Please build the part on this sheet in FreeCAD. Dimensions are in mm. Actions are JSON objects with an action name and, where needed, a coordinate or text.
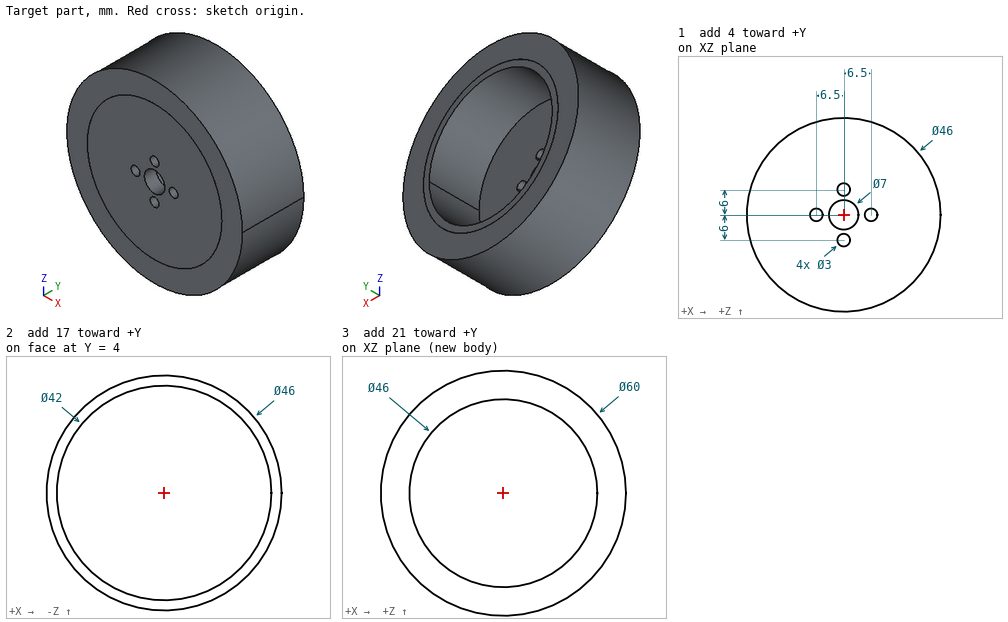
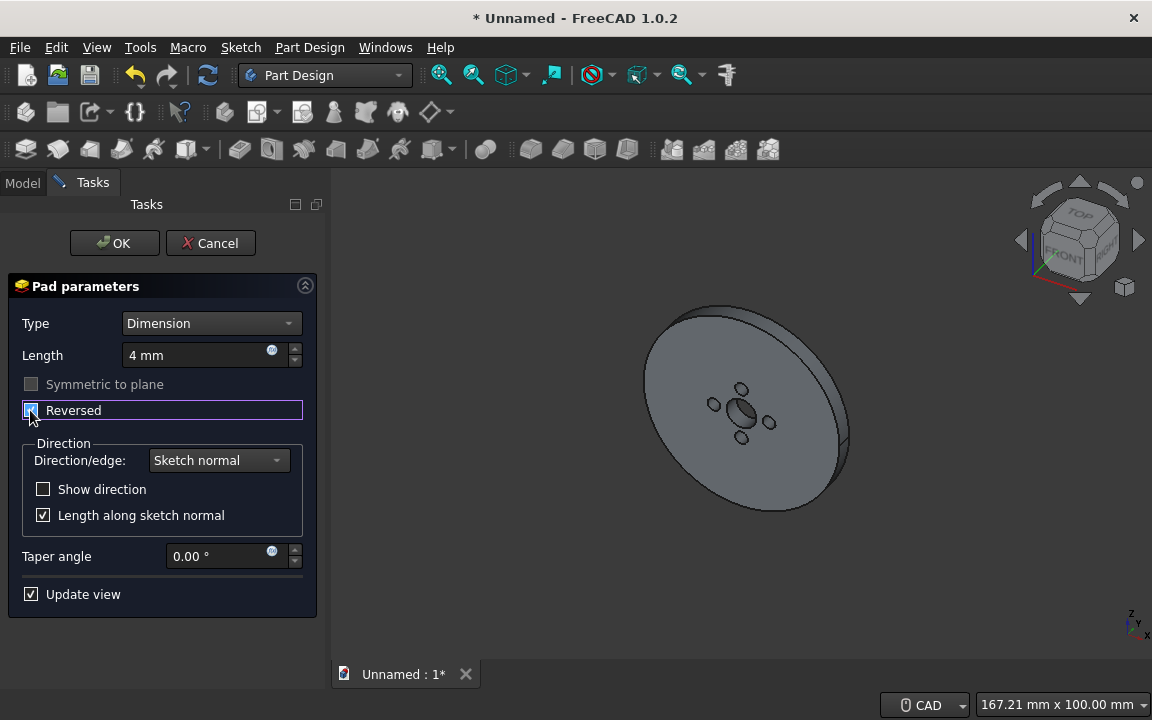
{"action": "left_click", "coordinate": [115, 243]}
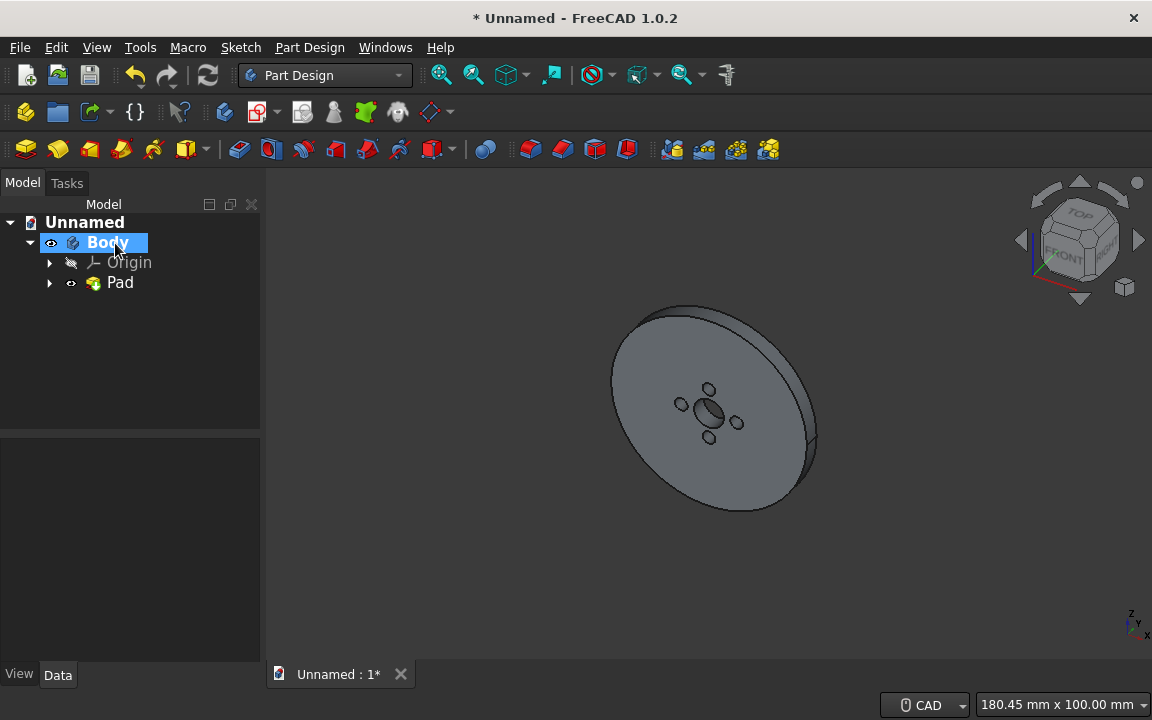
{"action": "key", "text": "4"}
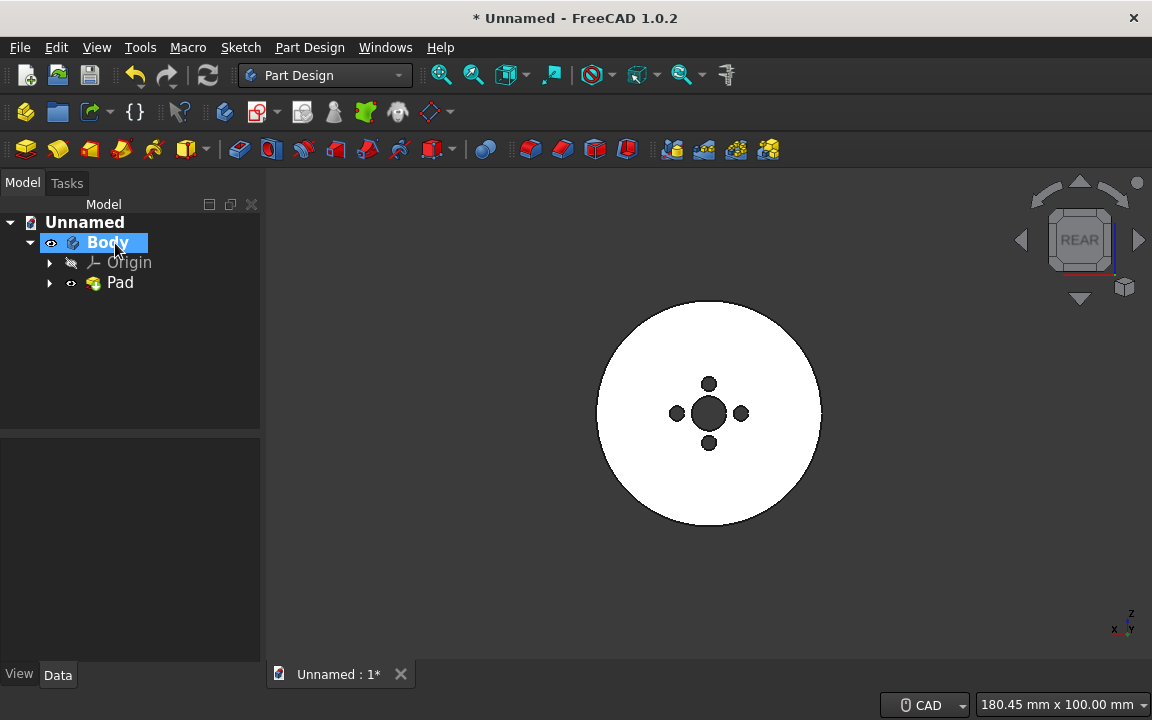
{"action": "left_click", "coordinate": [741, 348]}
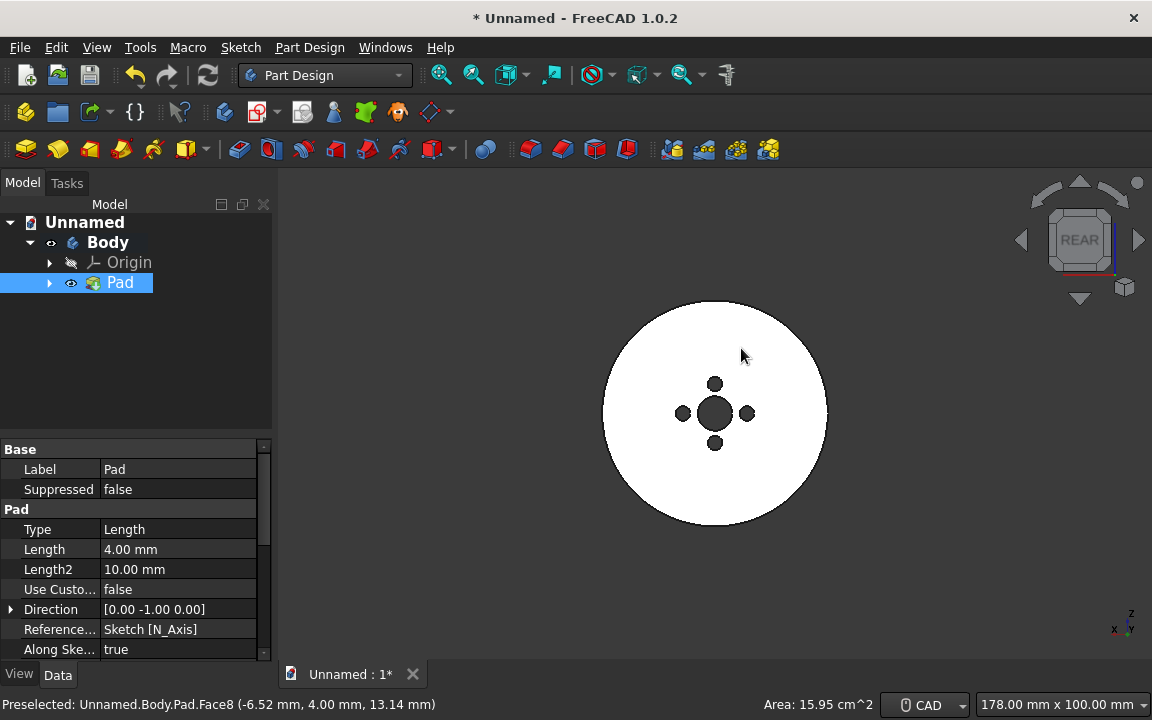
{"action": "left_click", "coordinate": [258, 112]}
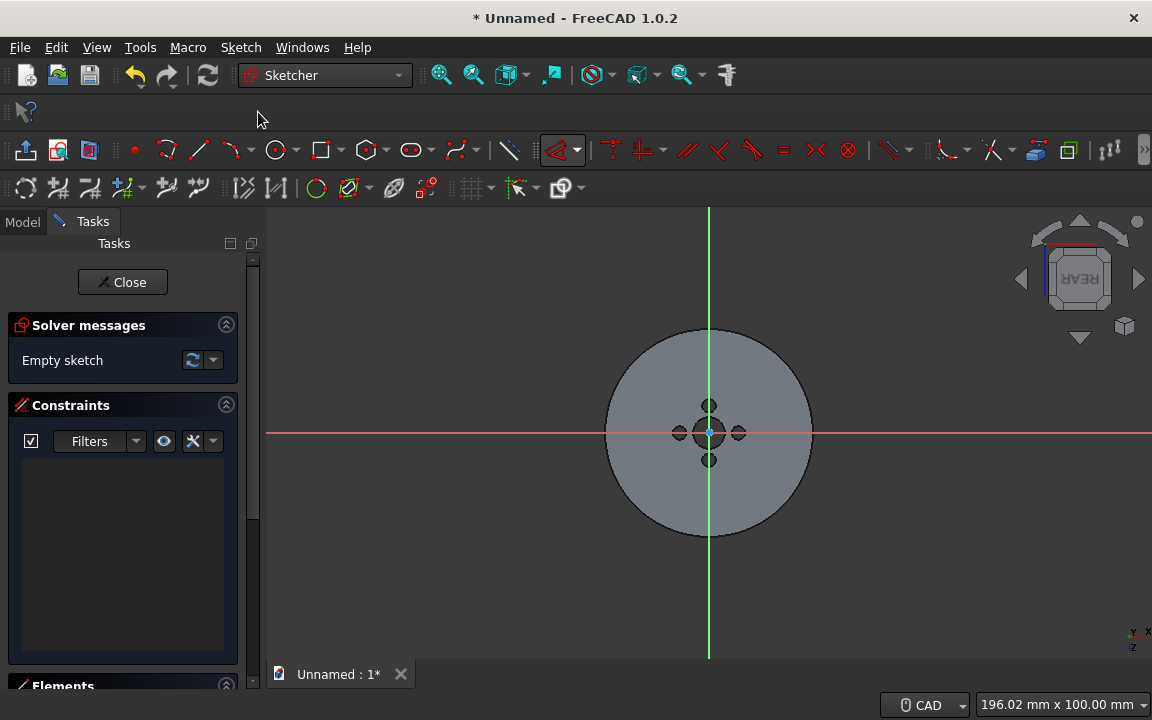
{"action": "left_click", "coordinate": [276, 150]}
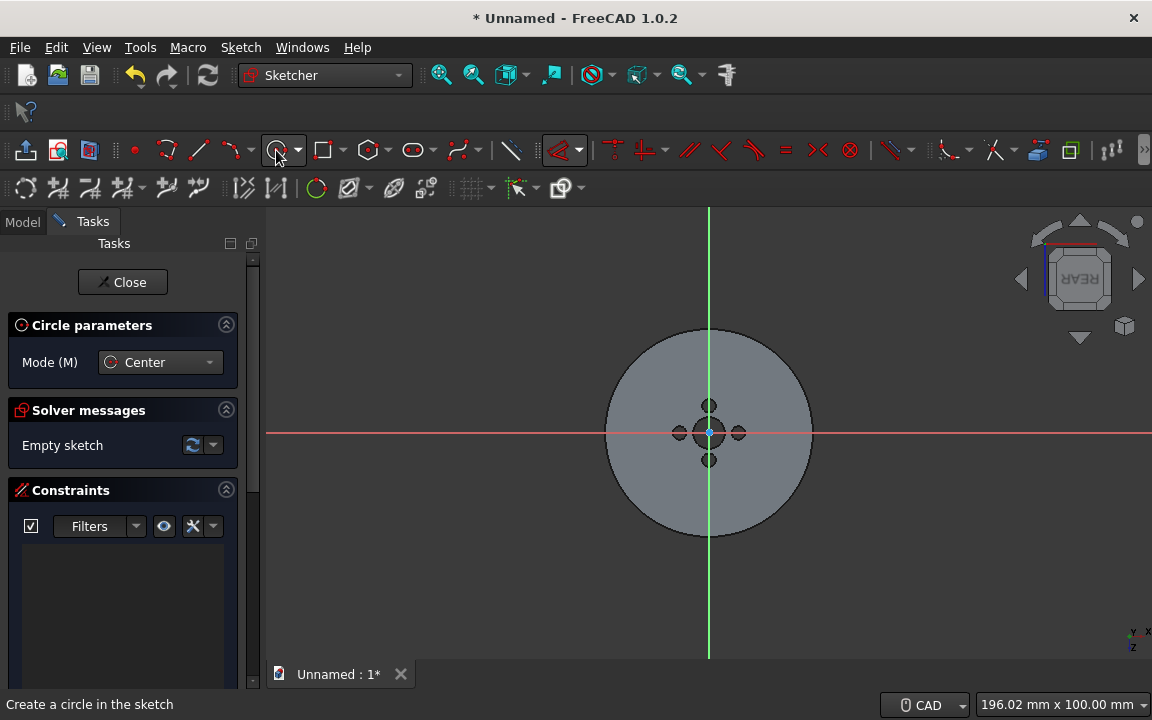
{"action": "left_click", "coordinate": [709, 433]}
{"action": "left_click", "coordinate": [783, 359]}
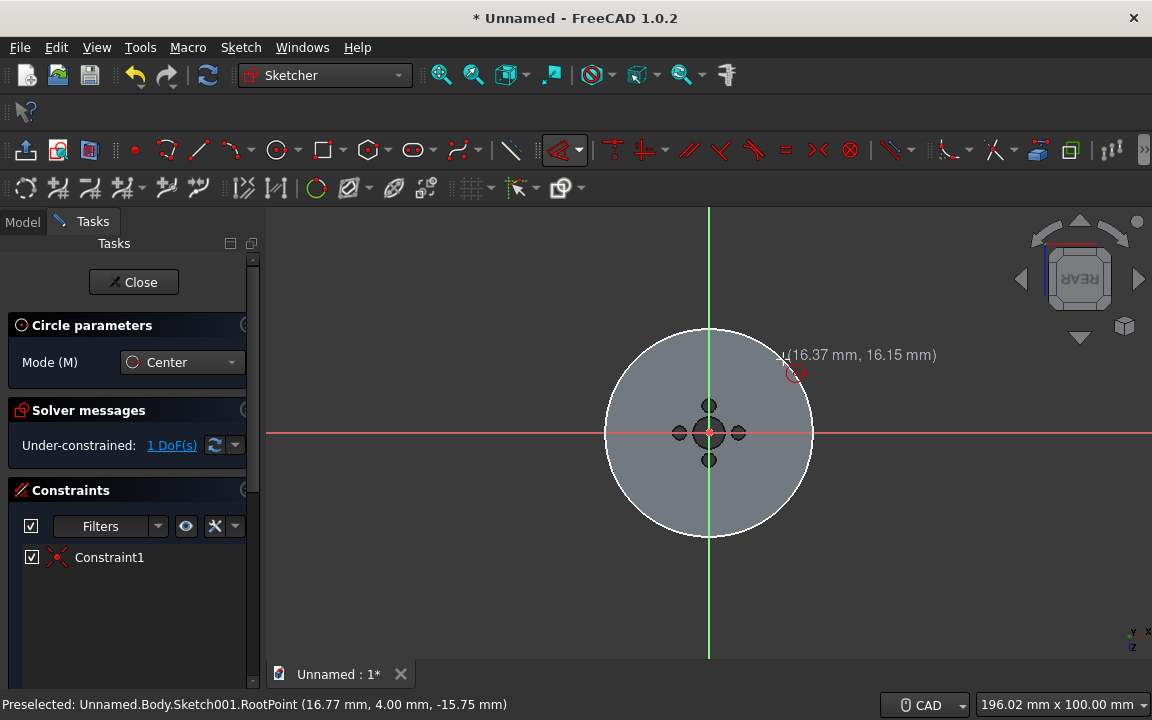
{"action": "left_click", "coordinate": [709, 433]}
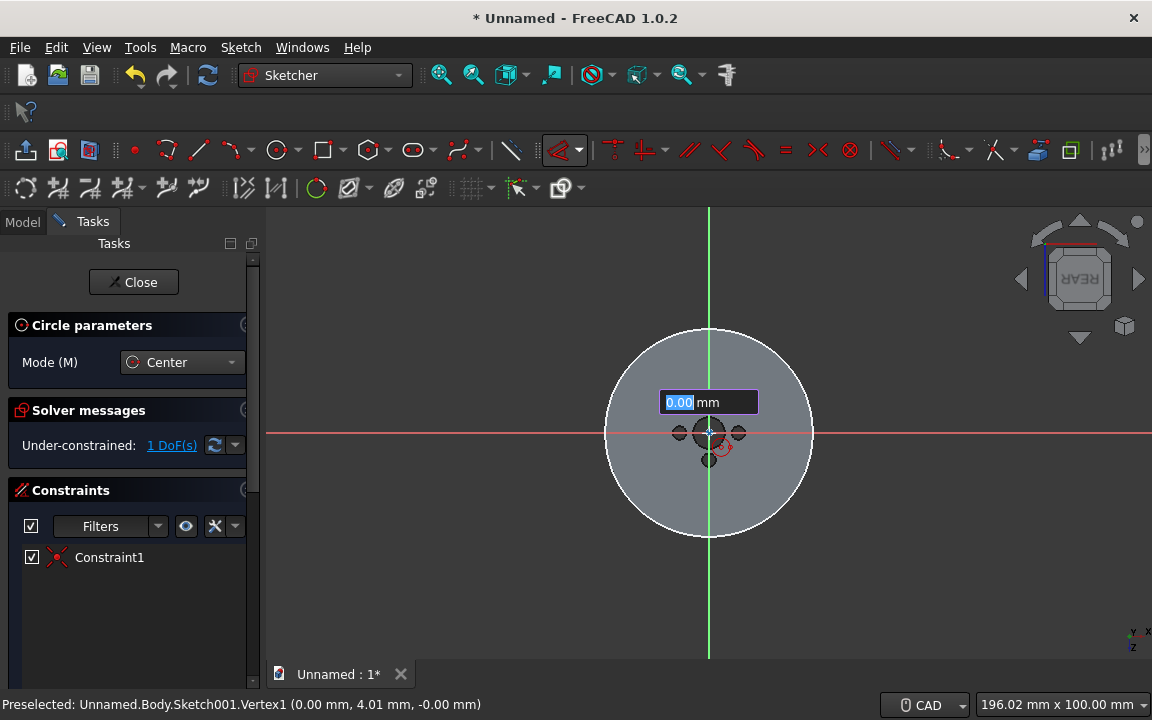
{"action": "scroll", "coordinate": [776, 366], "scroll_direction": "up", "scroll_amount": 3}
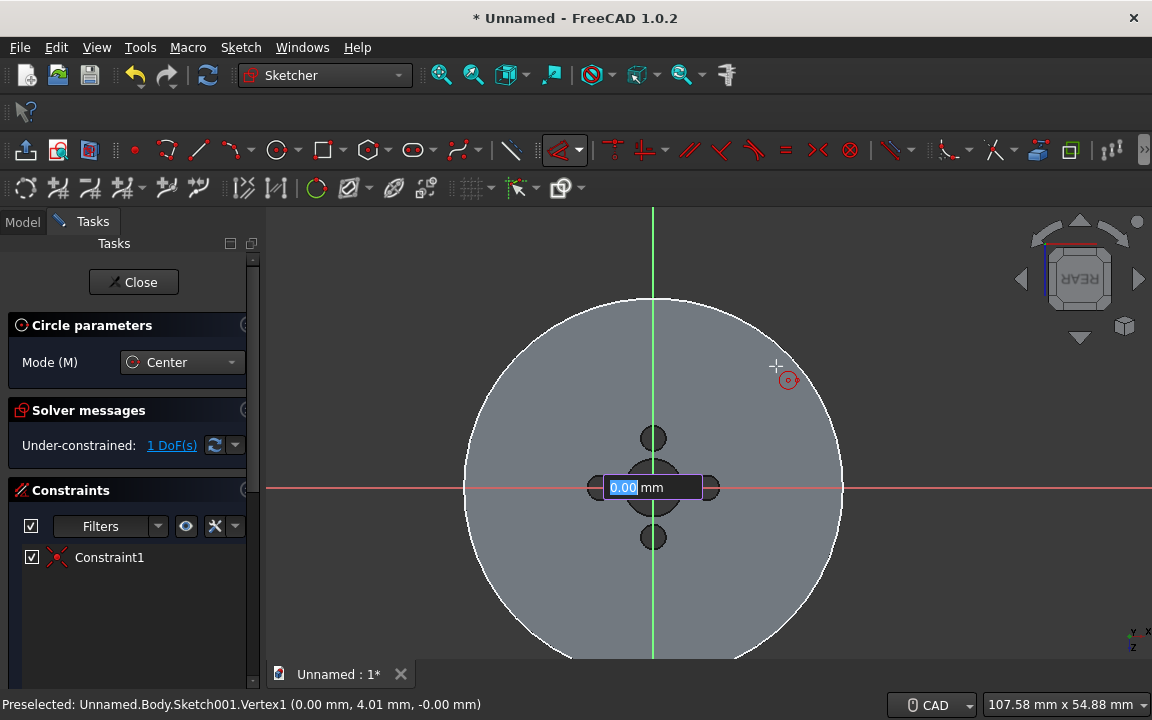
{"action": "left_click", "coordinate": [776, 365]}
{"action": "key", "text": "Escape"}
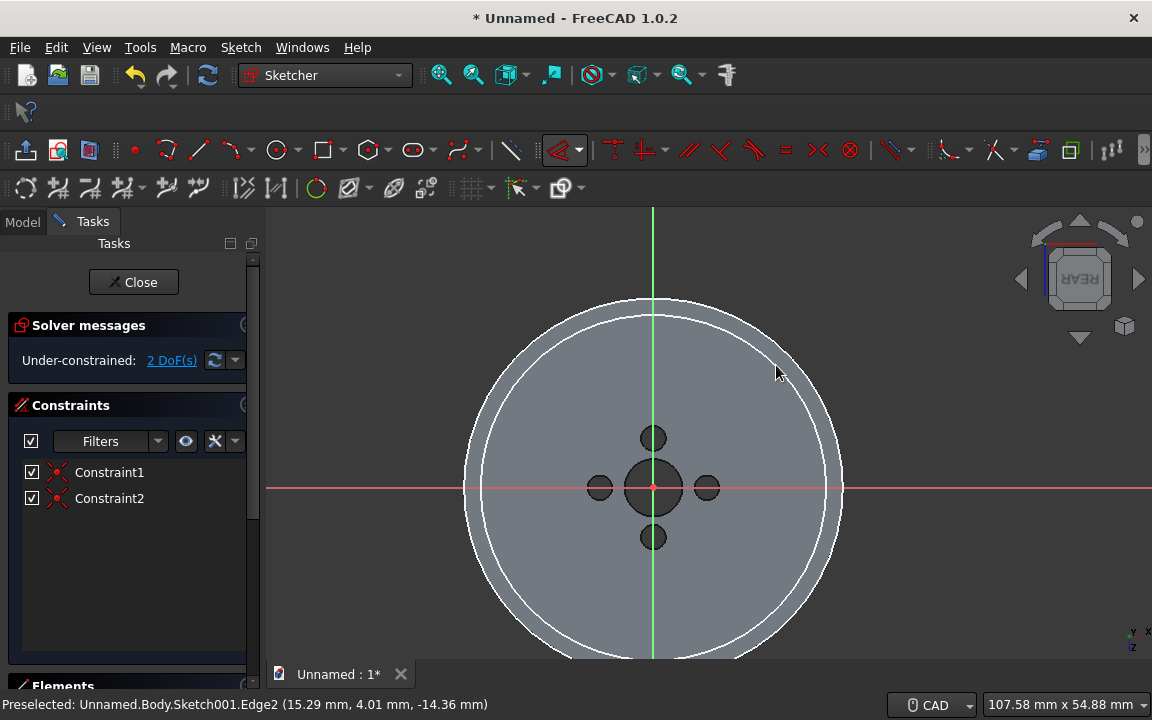
{"action": "left_click", "coordinate": [787, 353]}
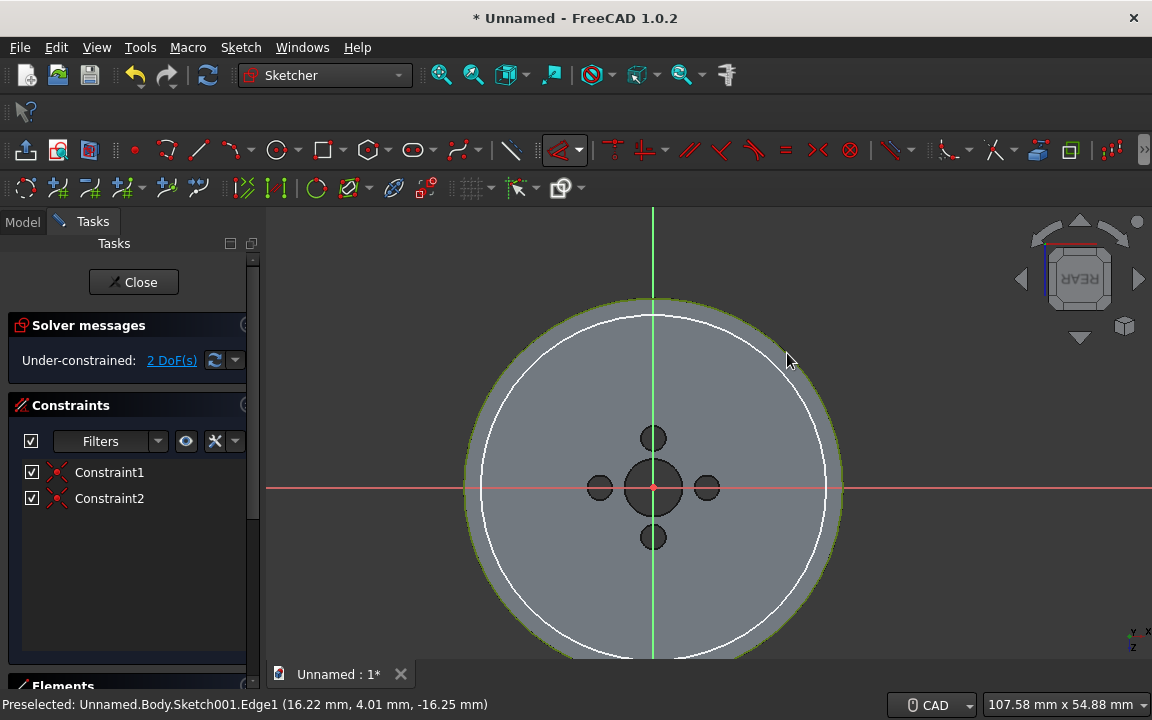
{"action": "key", "text": "k o"}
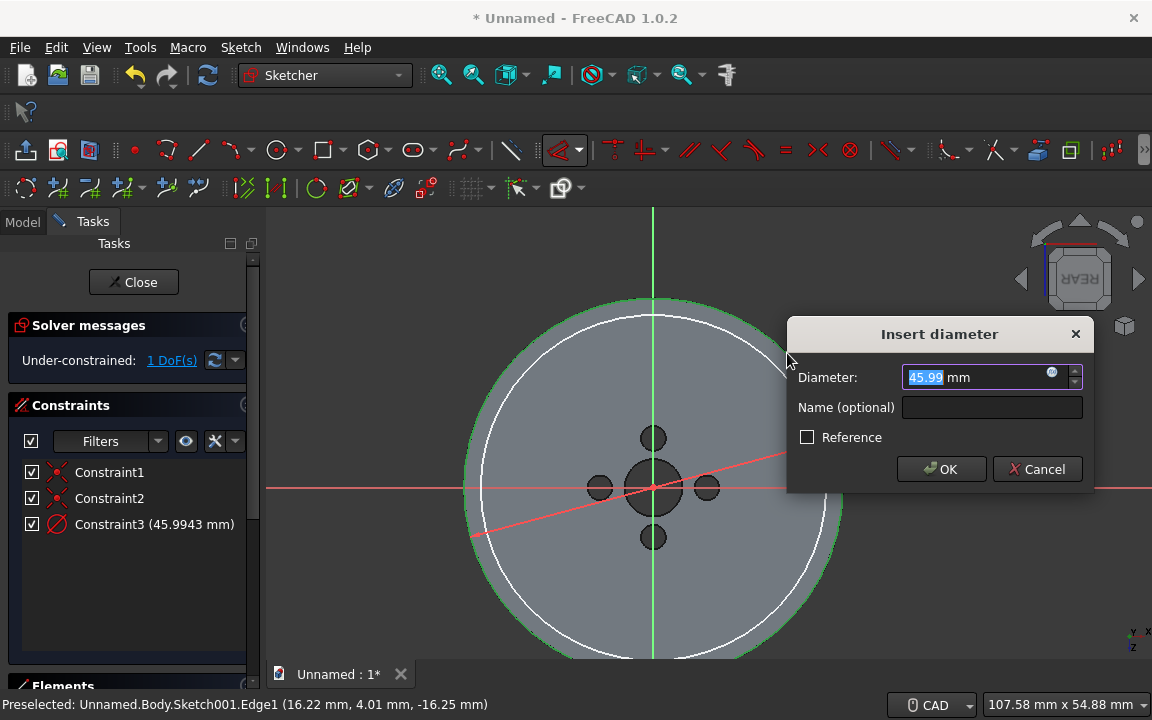
{"action": "type", "text": "46"}
{"action": "key", "text": "Return"}